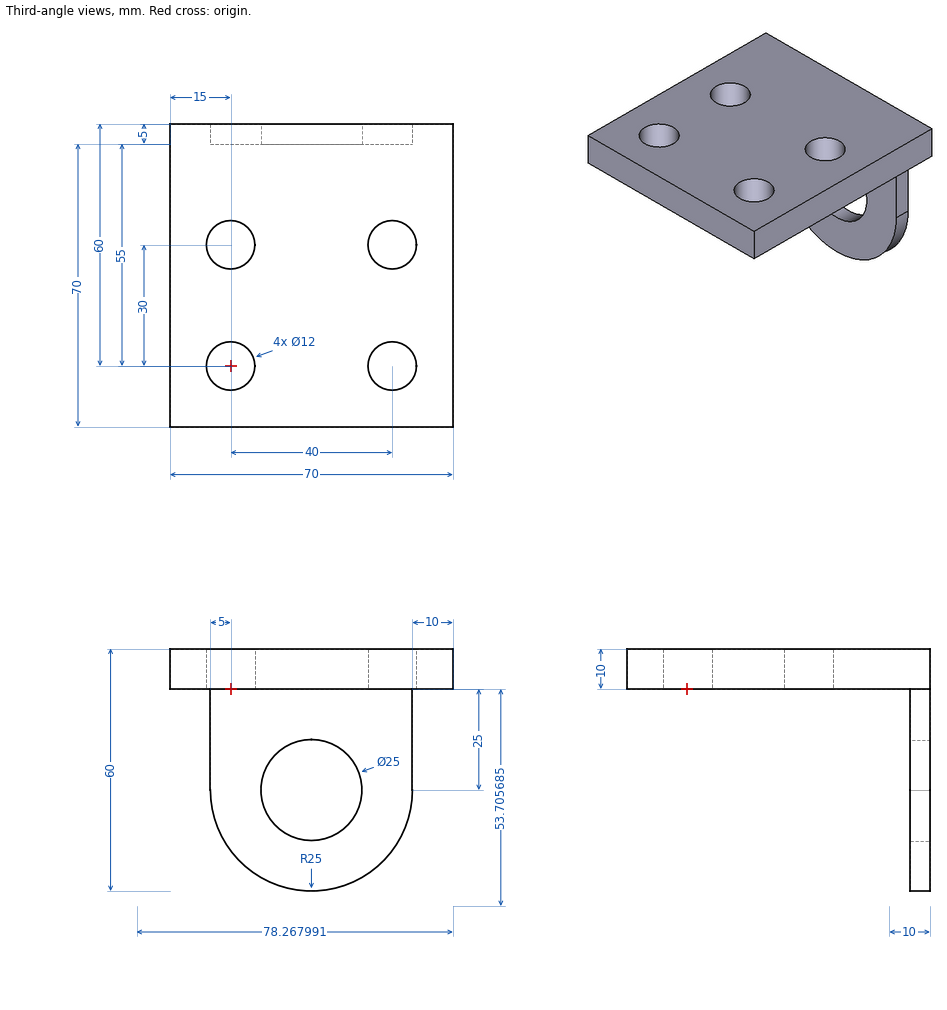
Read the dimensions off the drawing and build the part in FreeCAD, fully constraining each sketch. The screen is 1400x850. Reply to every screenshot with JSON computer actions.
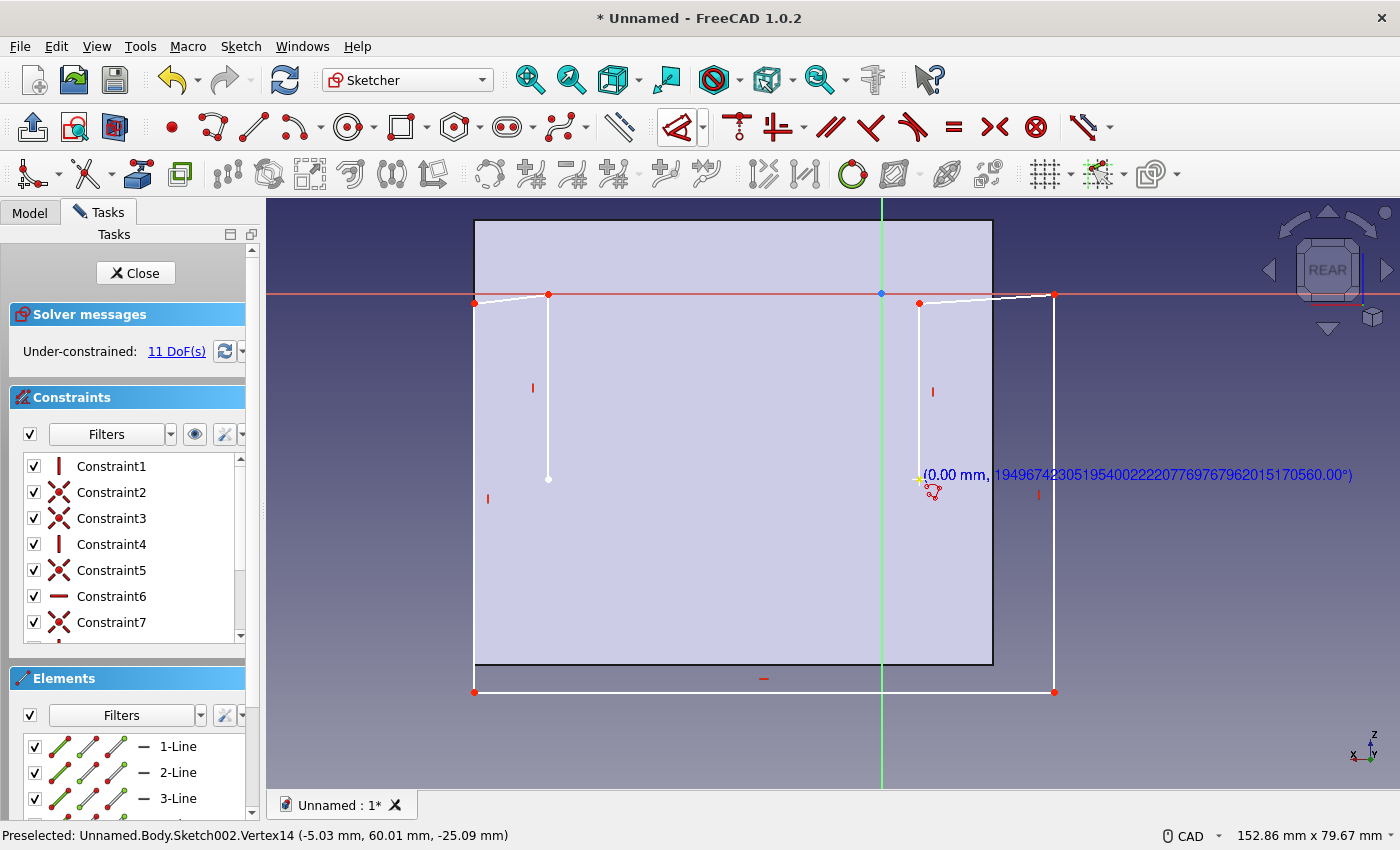
{"action": "key", "text": "g 3 a"}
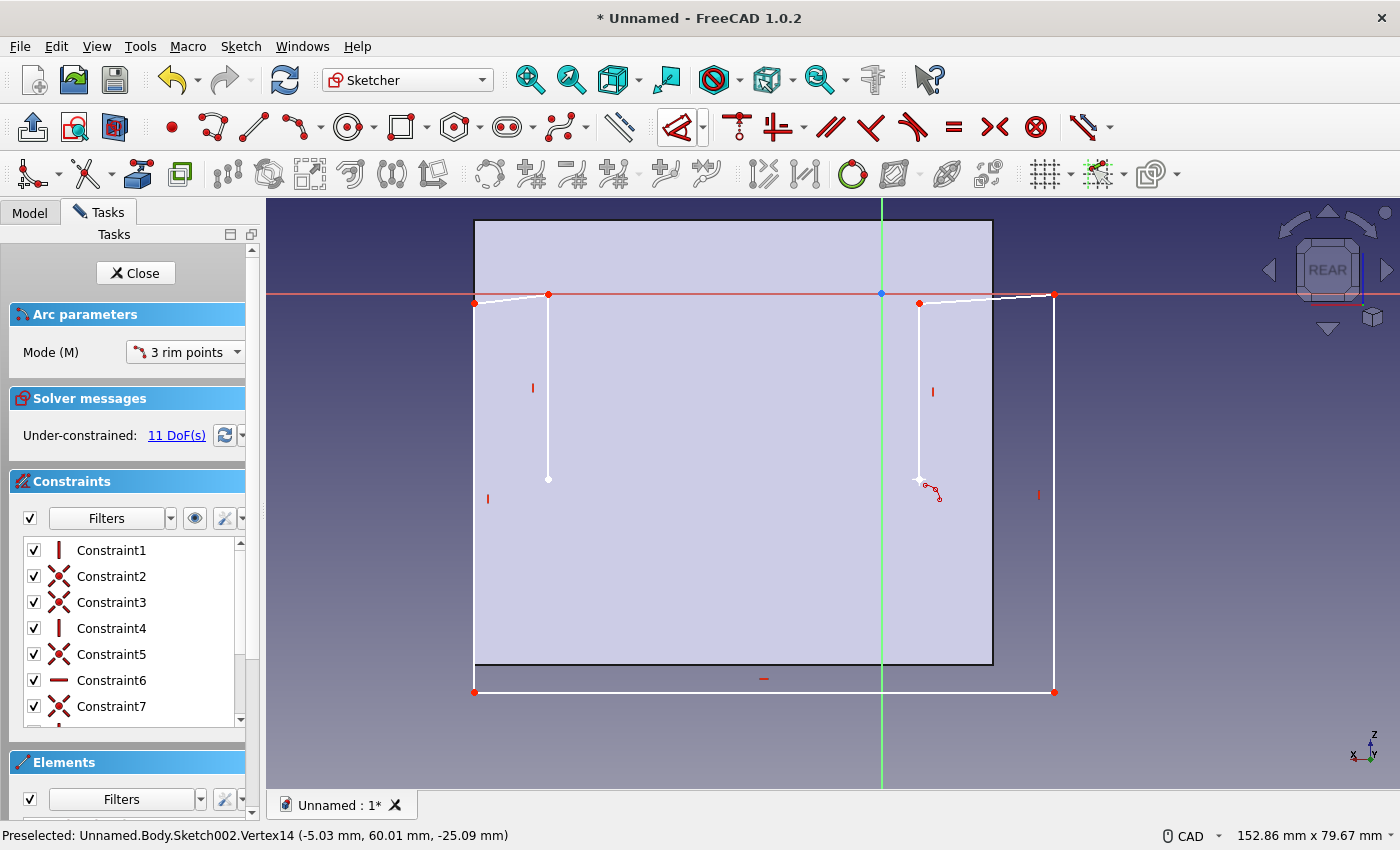
{"action": "left_click", "coordinate": [919, 480]}
{"action": "left_click", "coordinate": [548, 480]}
{"action": "left_click", "coordinate": [733, 665]}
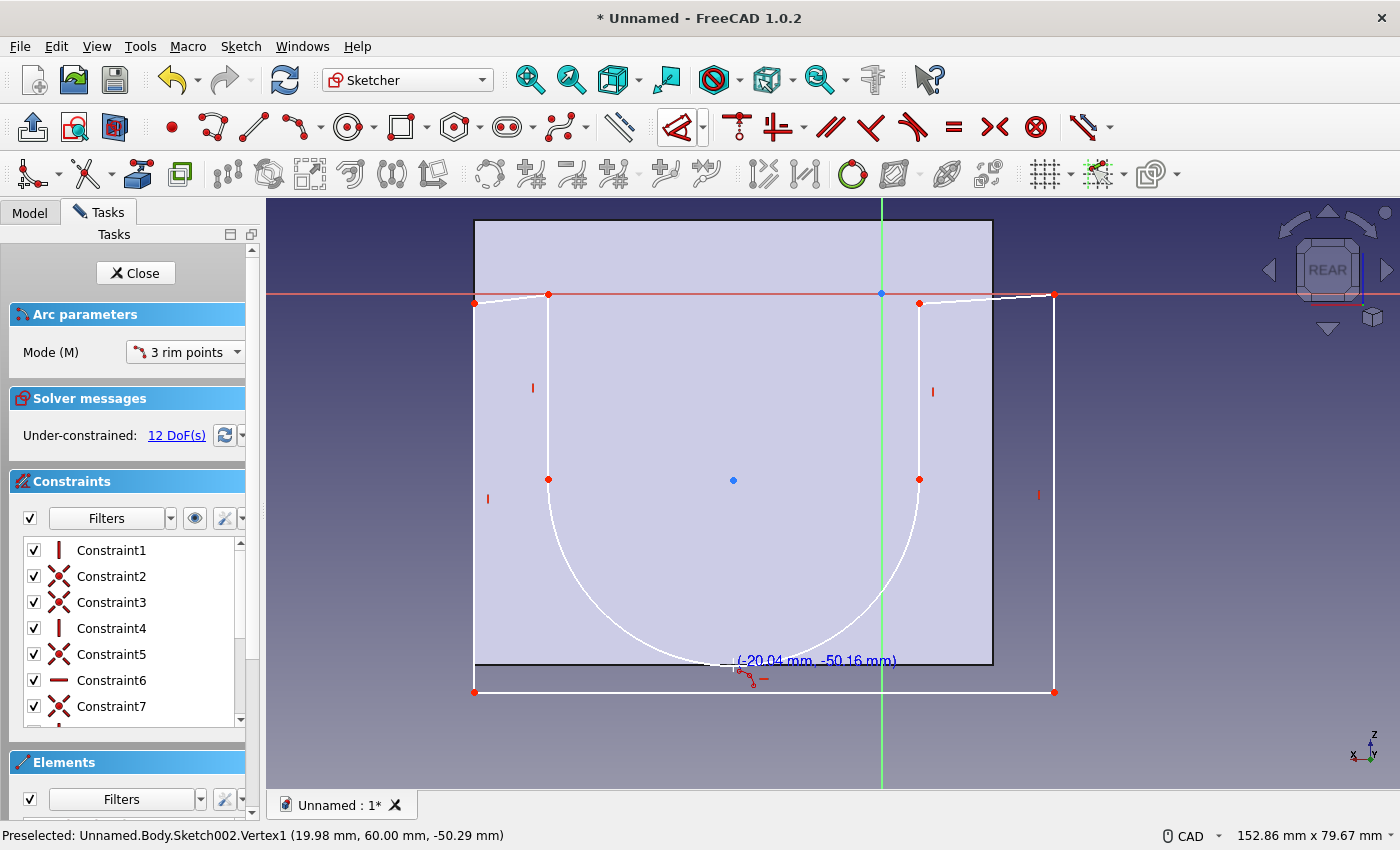
{"action": "left_click", "coordinate": [348, 128]}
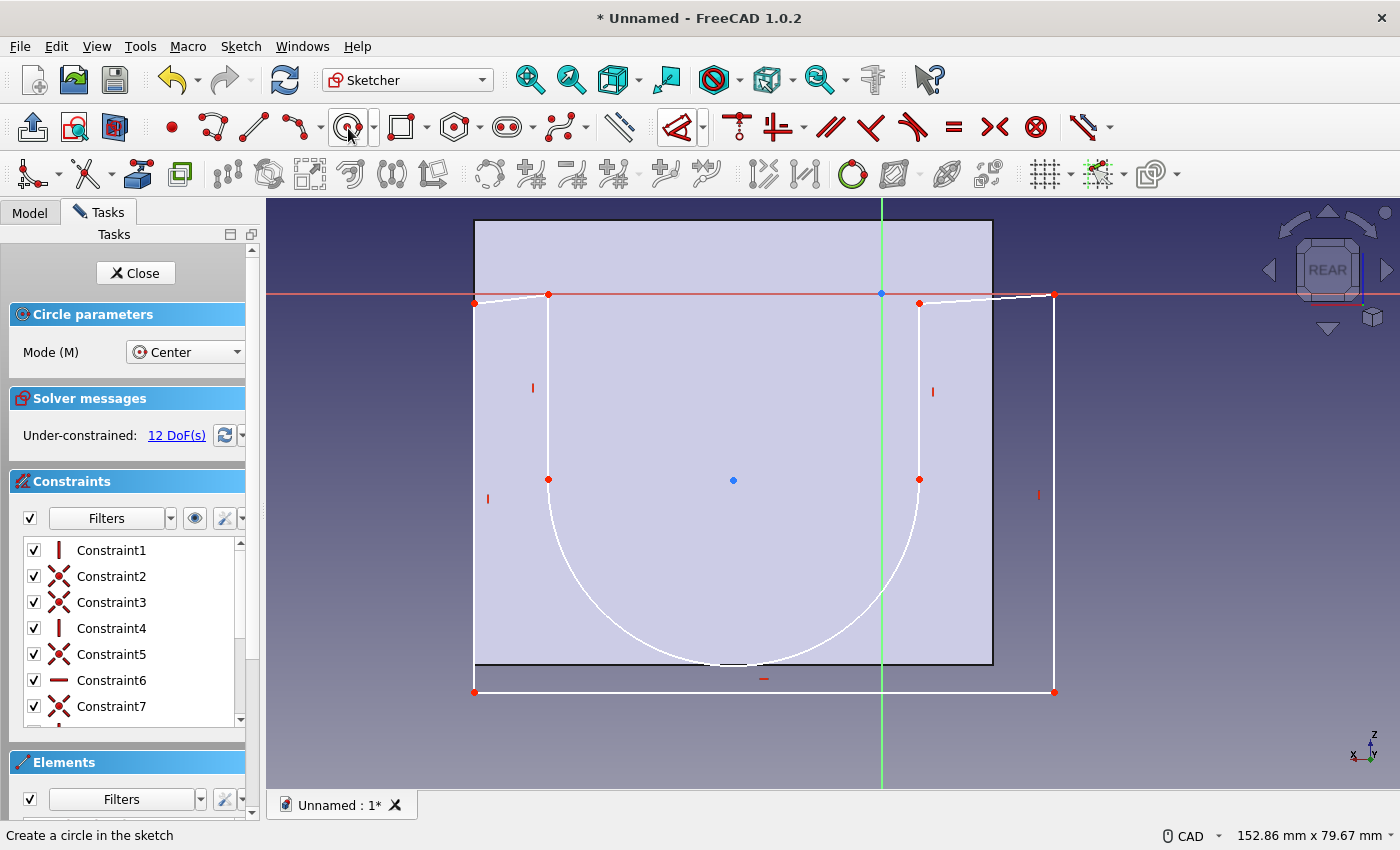
{"action": "left_click", "coordinate": [733, 479]}
{"action": "left_click", "coordinate": [799, 414]}
{"action": "key", "text": "Escape"}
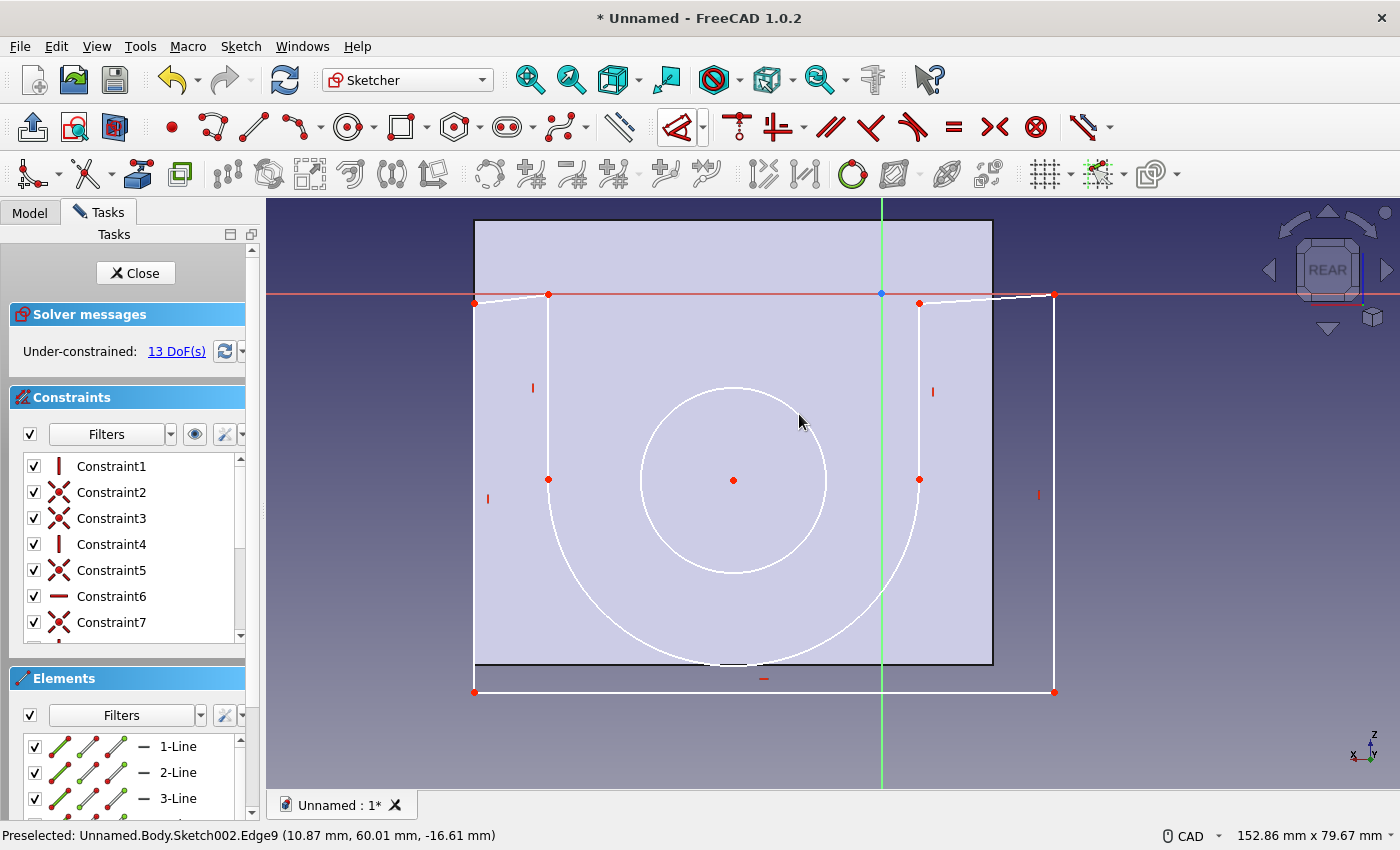
{"action": "left_click", "coordinate": [548, 425]}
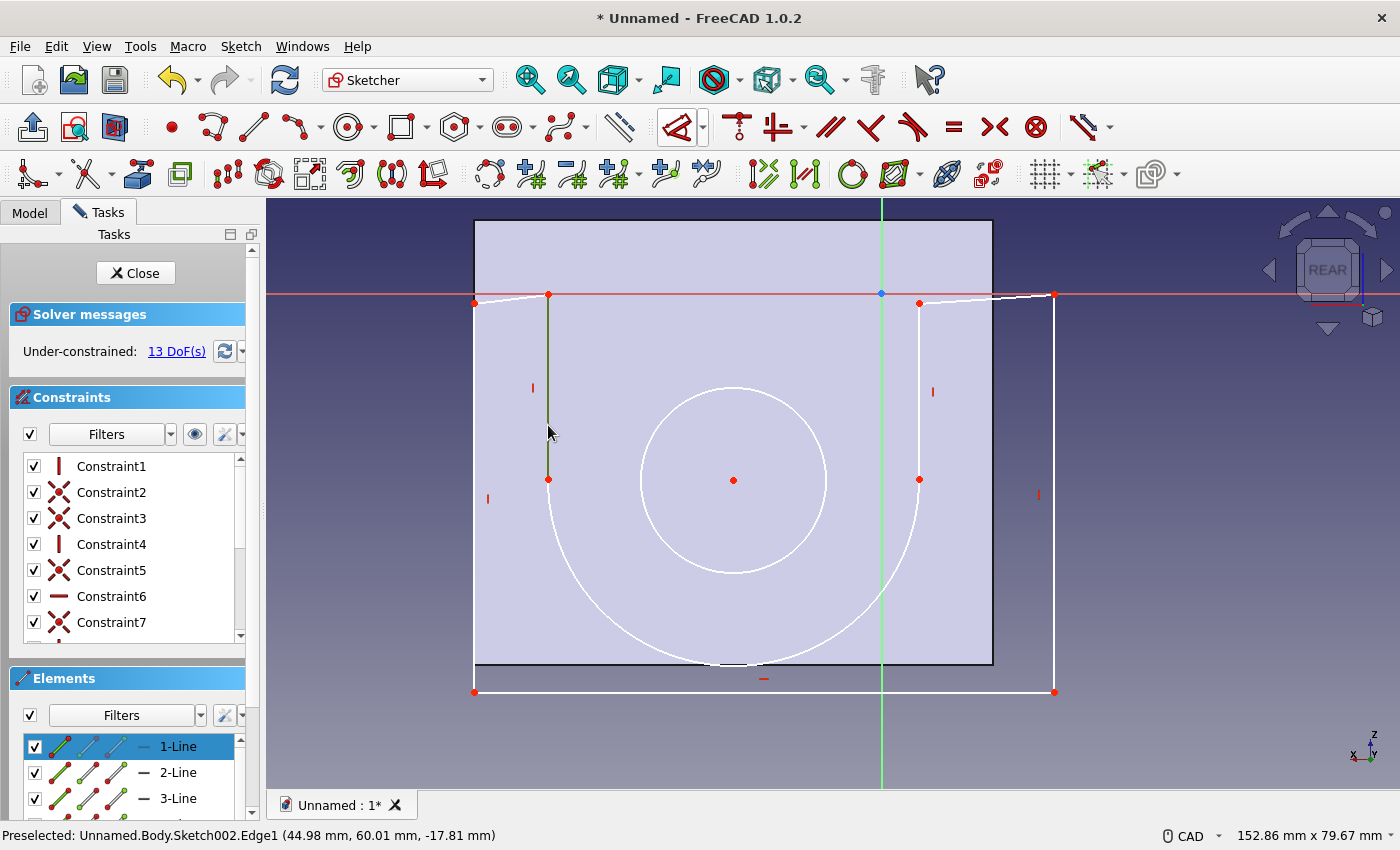
{"action": "left_click", "coordinate": [624, 630]}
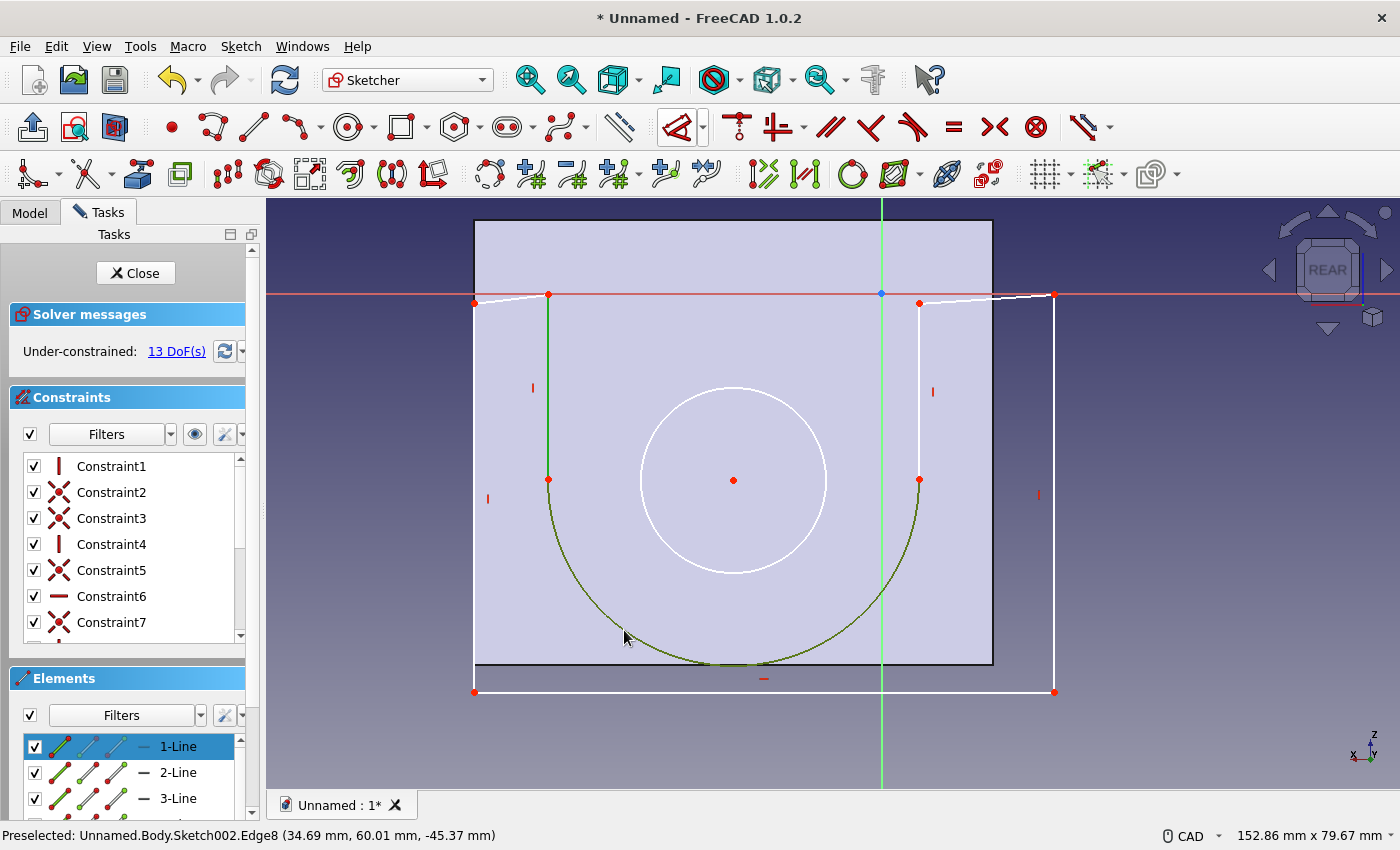
{"action": "left_click", "coordinate": [913, 128]}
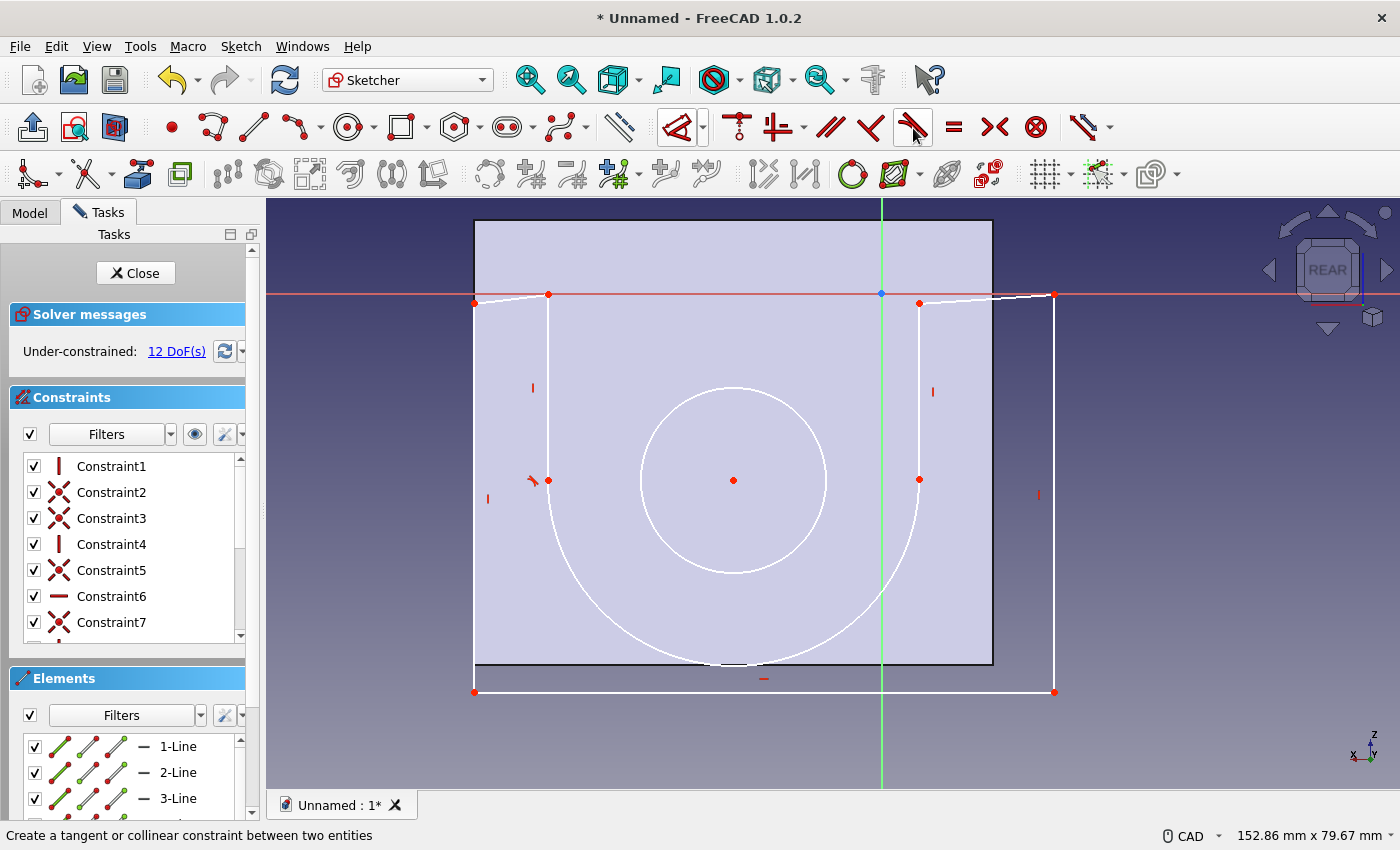
{"action": "left_click", "coordinate": [919, 357]}